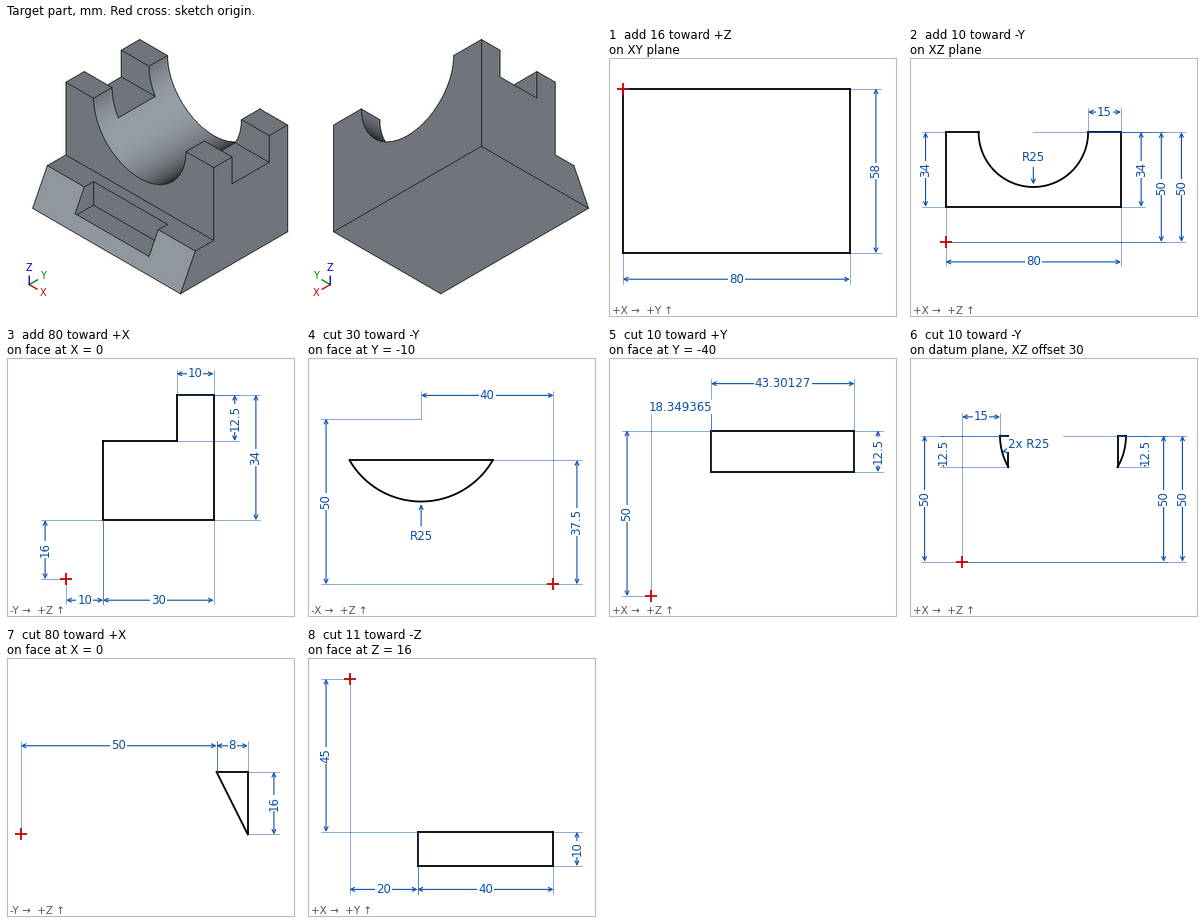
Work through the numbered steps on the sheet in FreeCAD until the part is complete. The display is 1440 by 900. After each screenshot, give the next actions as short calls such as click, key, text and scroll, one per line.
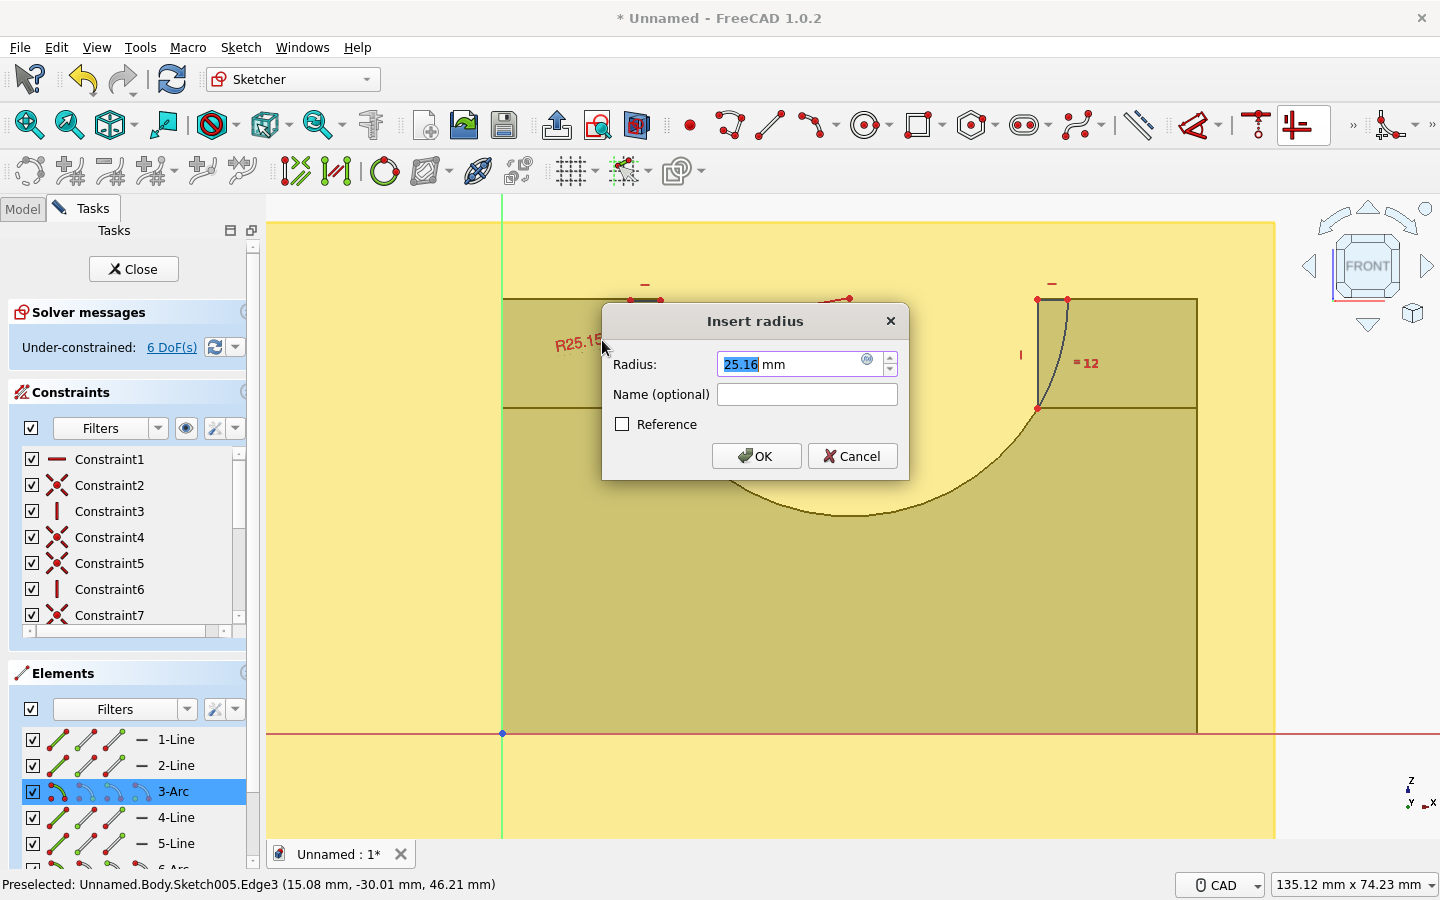
text(25)
key(Return)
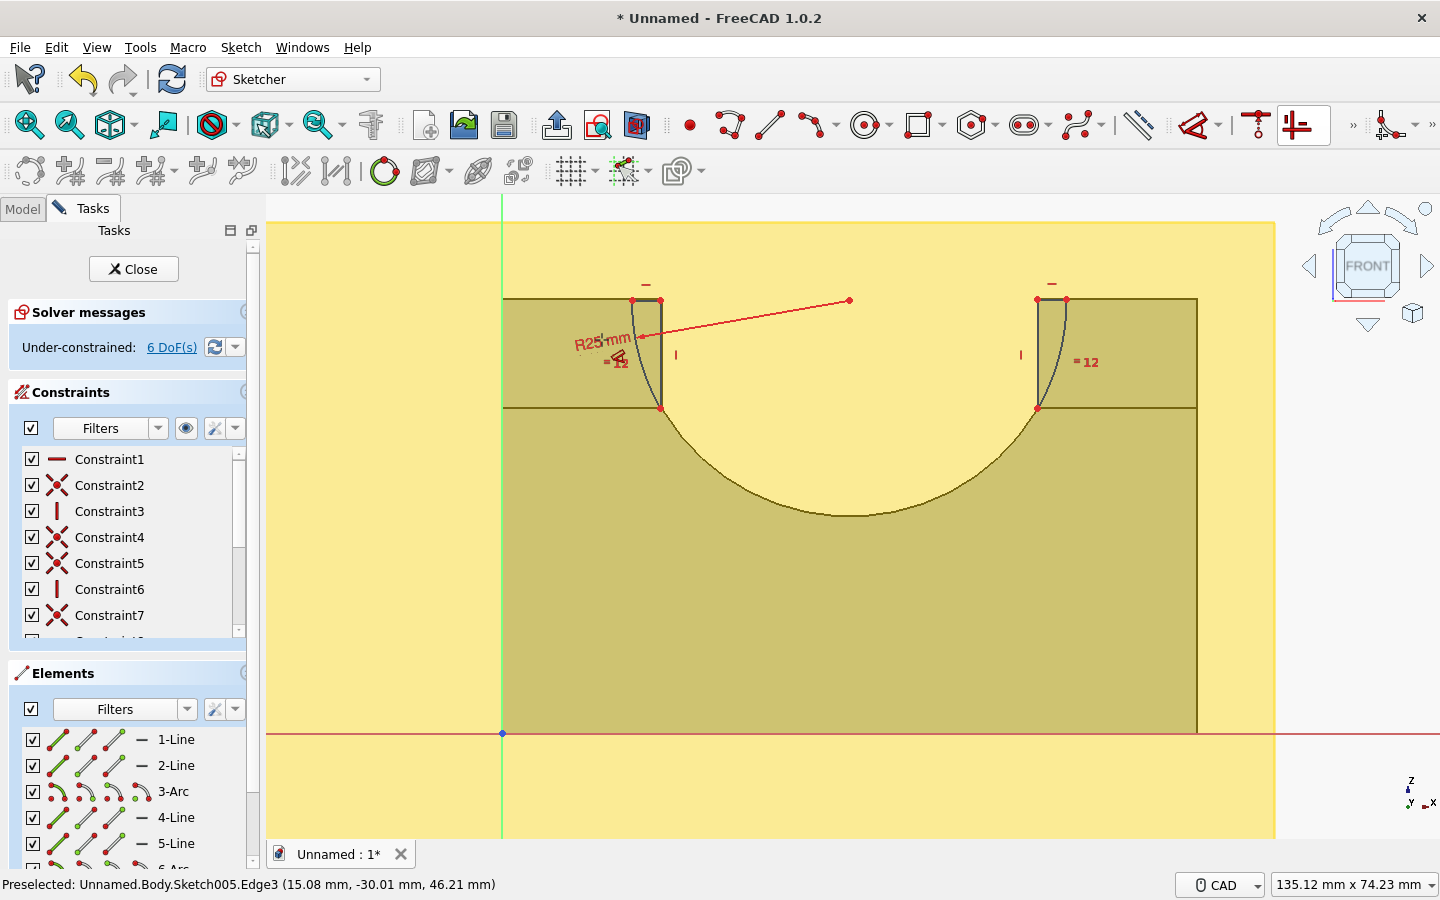
click(632, 301)
click(567, 768)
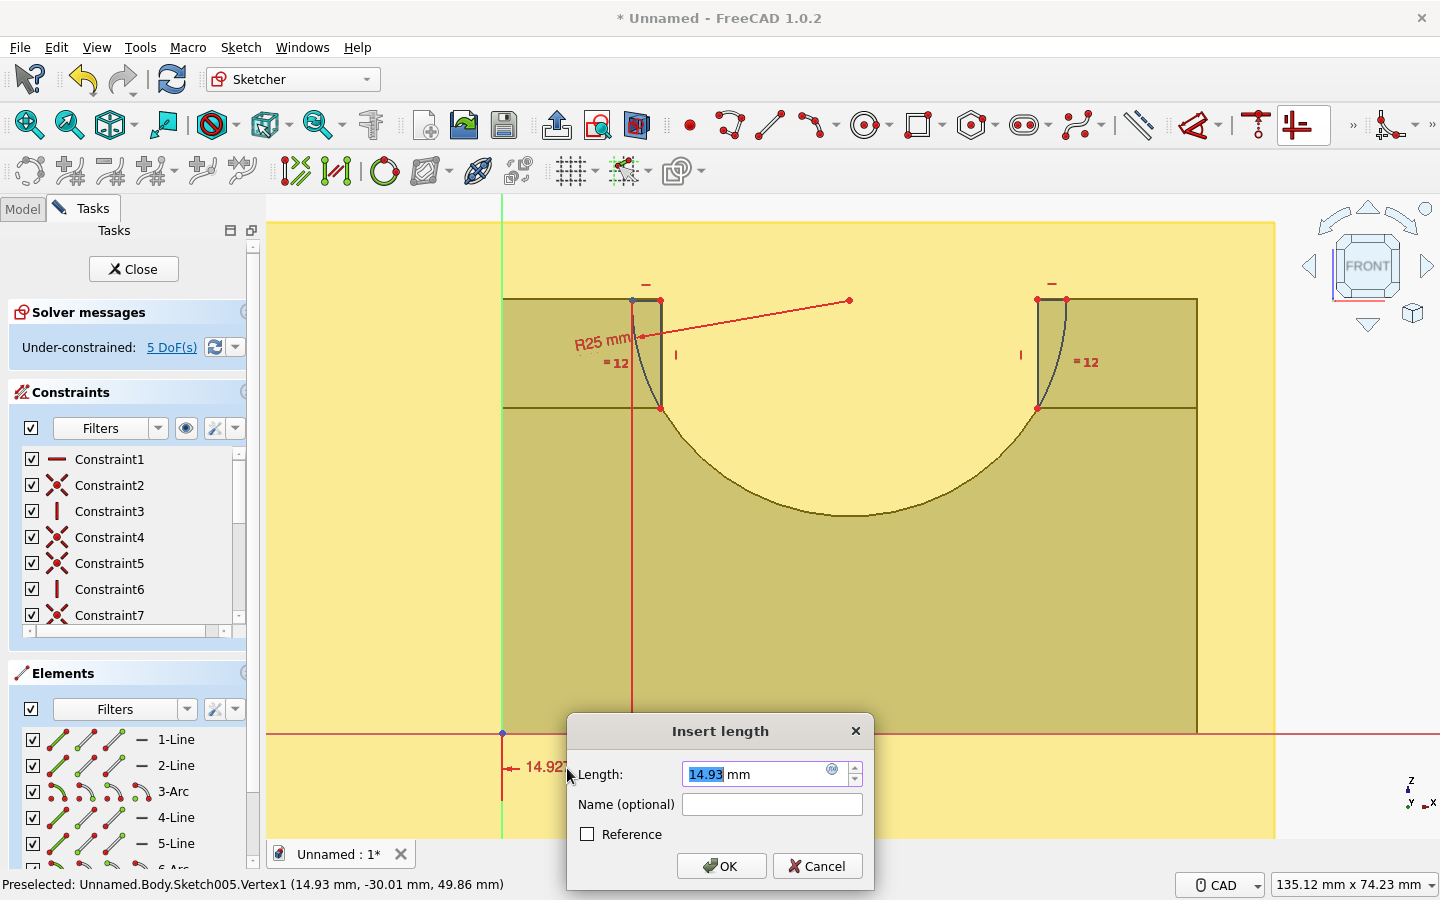
text(15)
key(Return)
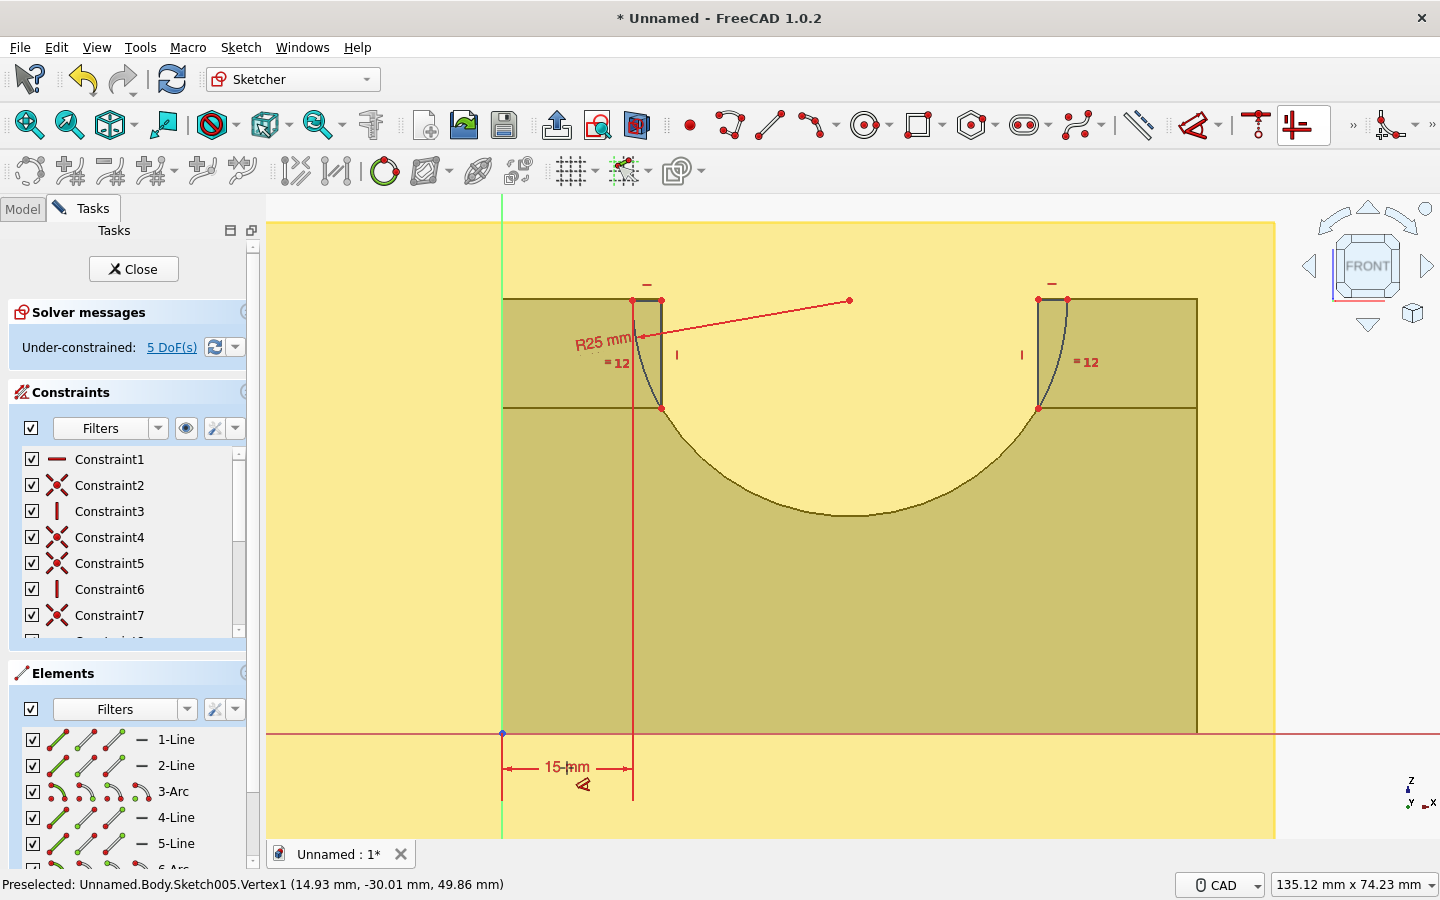
click(633, 301)
click(468, 517)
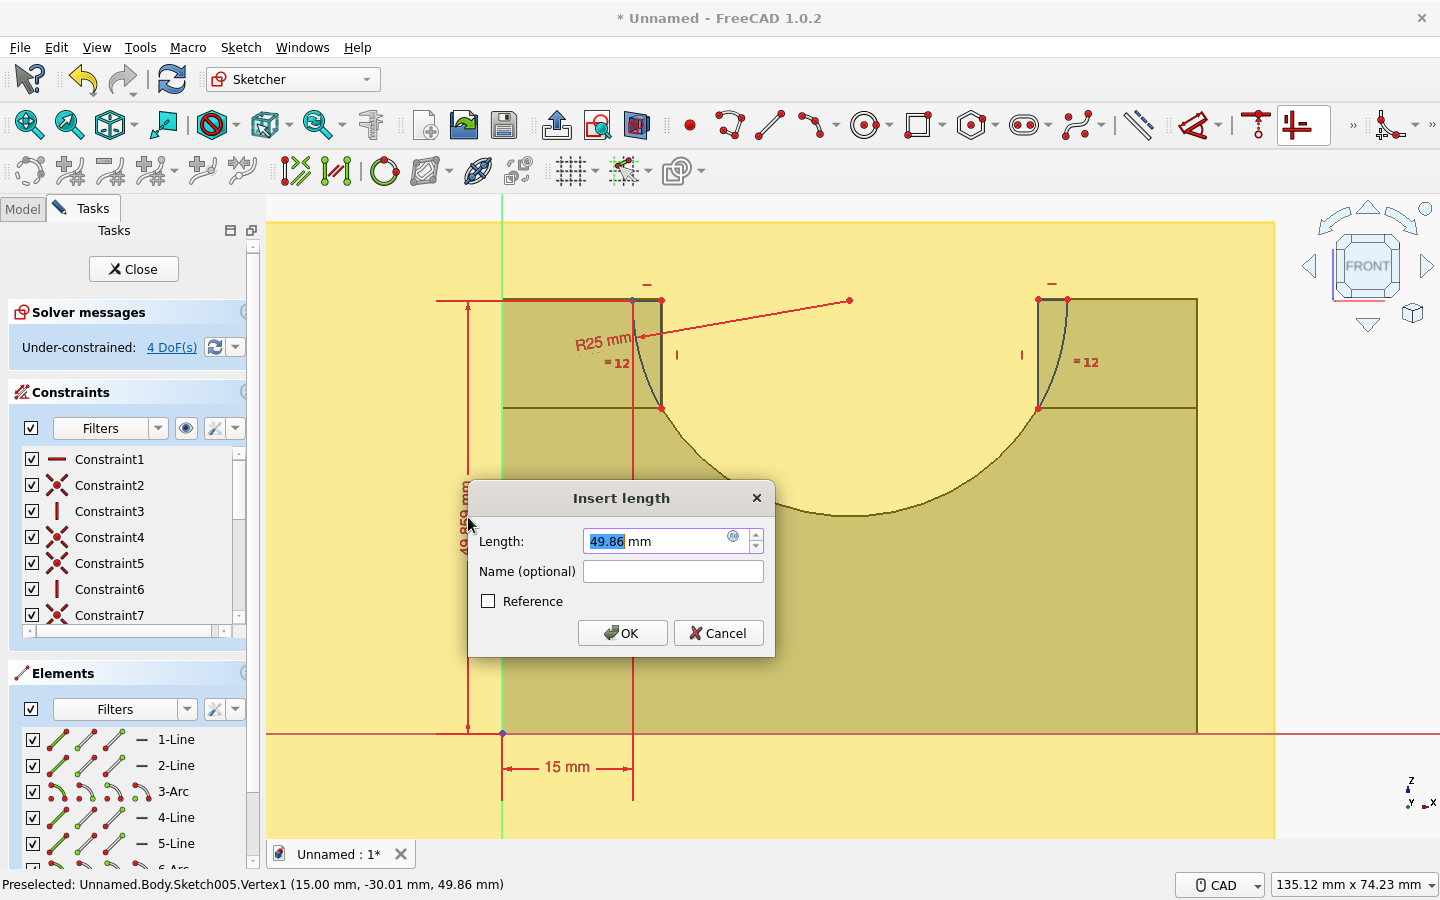
text(50)
key(Return)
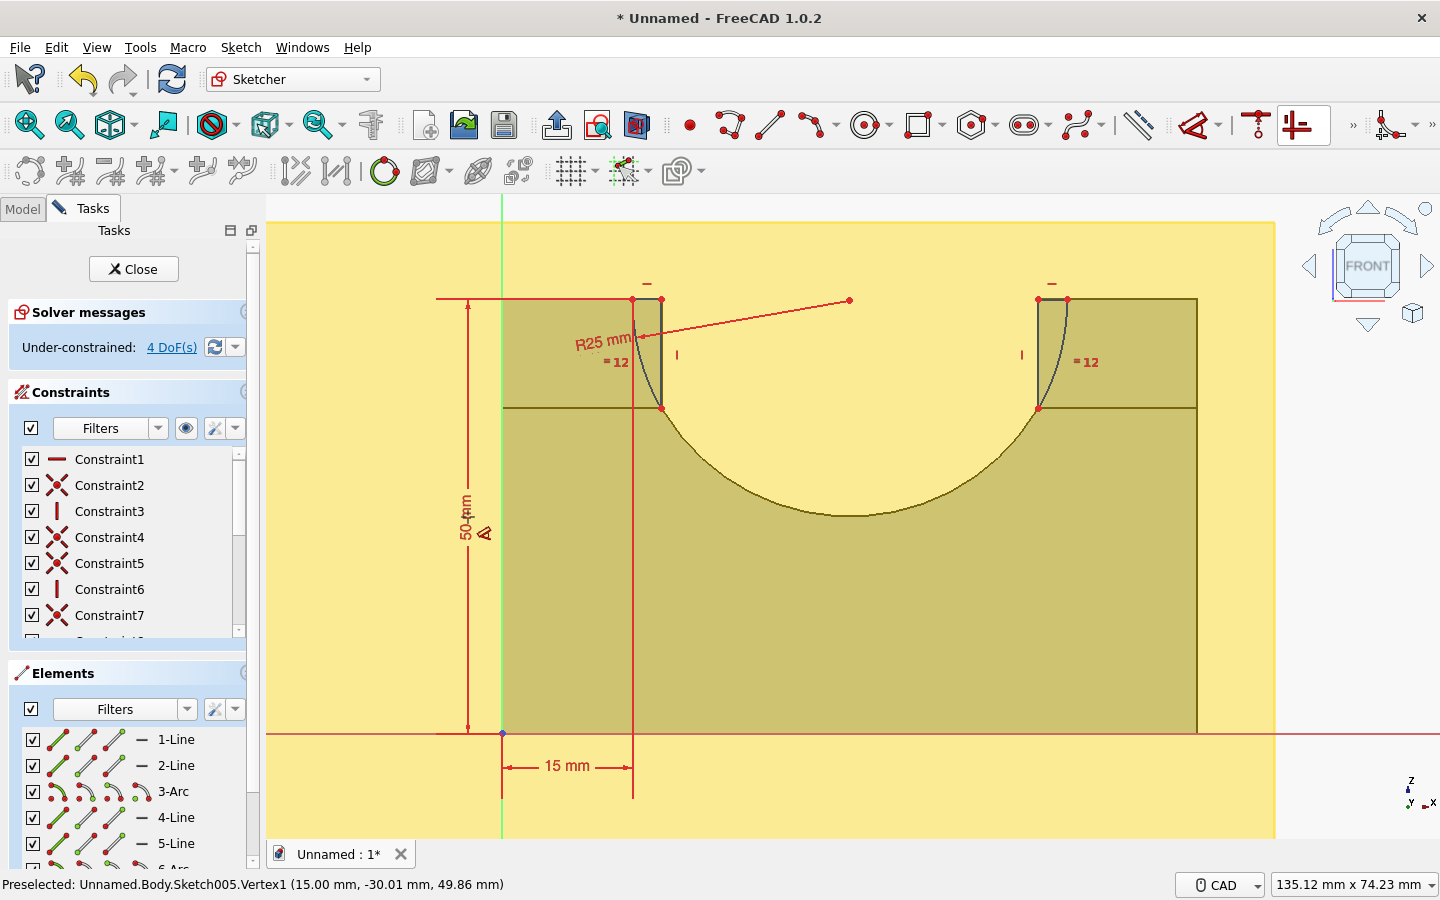
click(1038, 300)
click(468, 417)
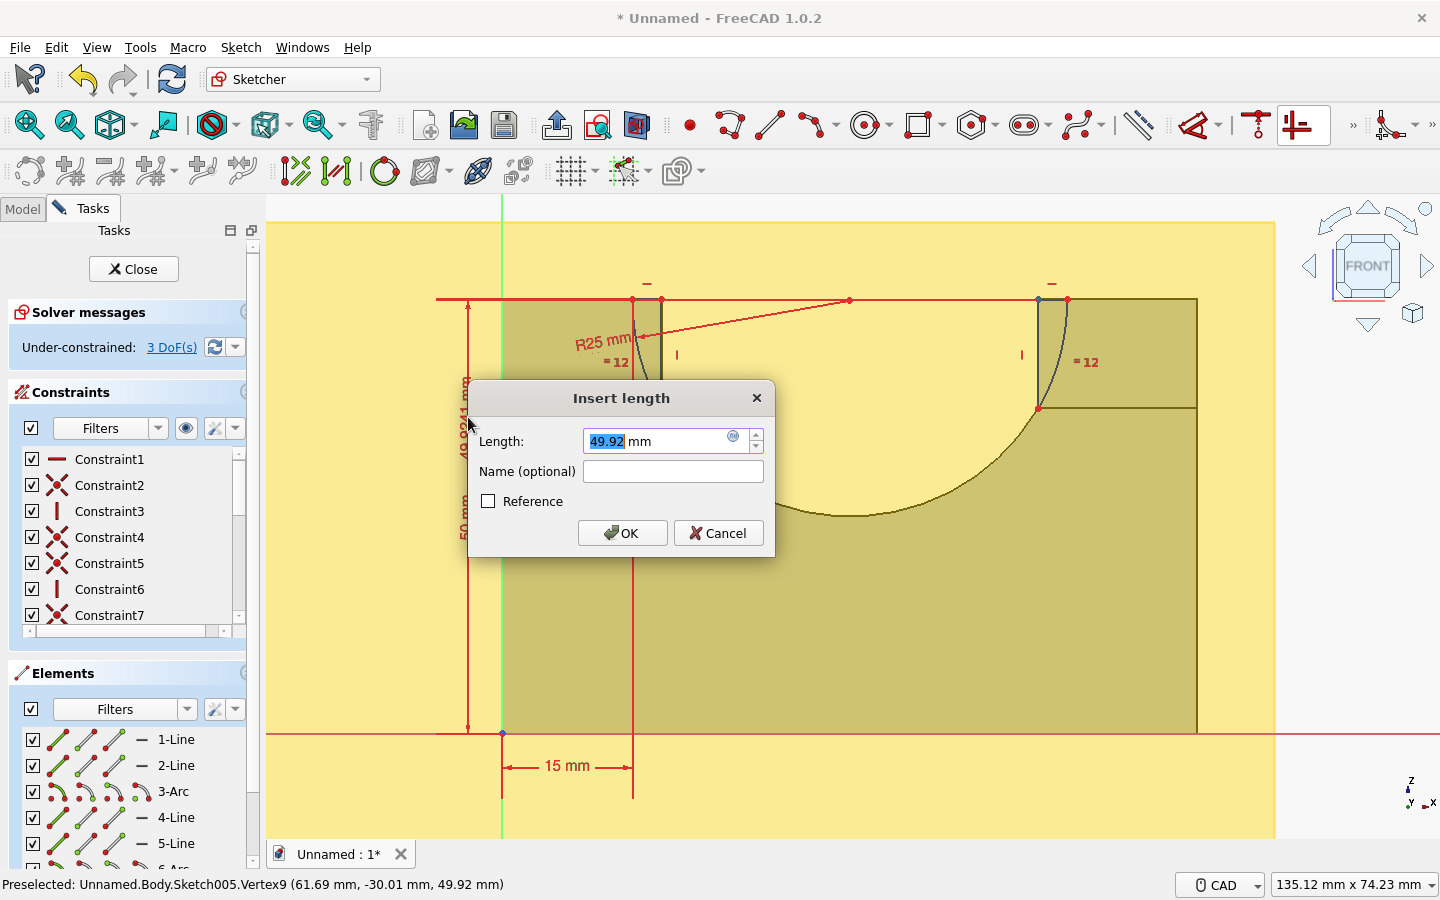
text(50)
key(Return)